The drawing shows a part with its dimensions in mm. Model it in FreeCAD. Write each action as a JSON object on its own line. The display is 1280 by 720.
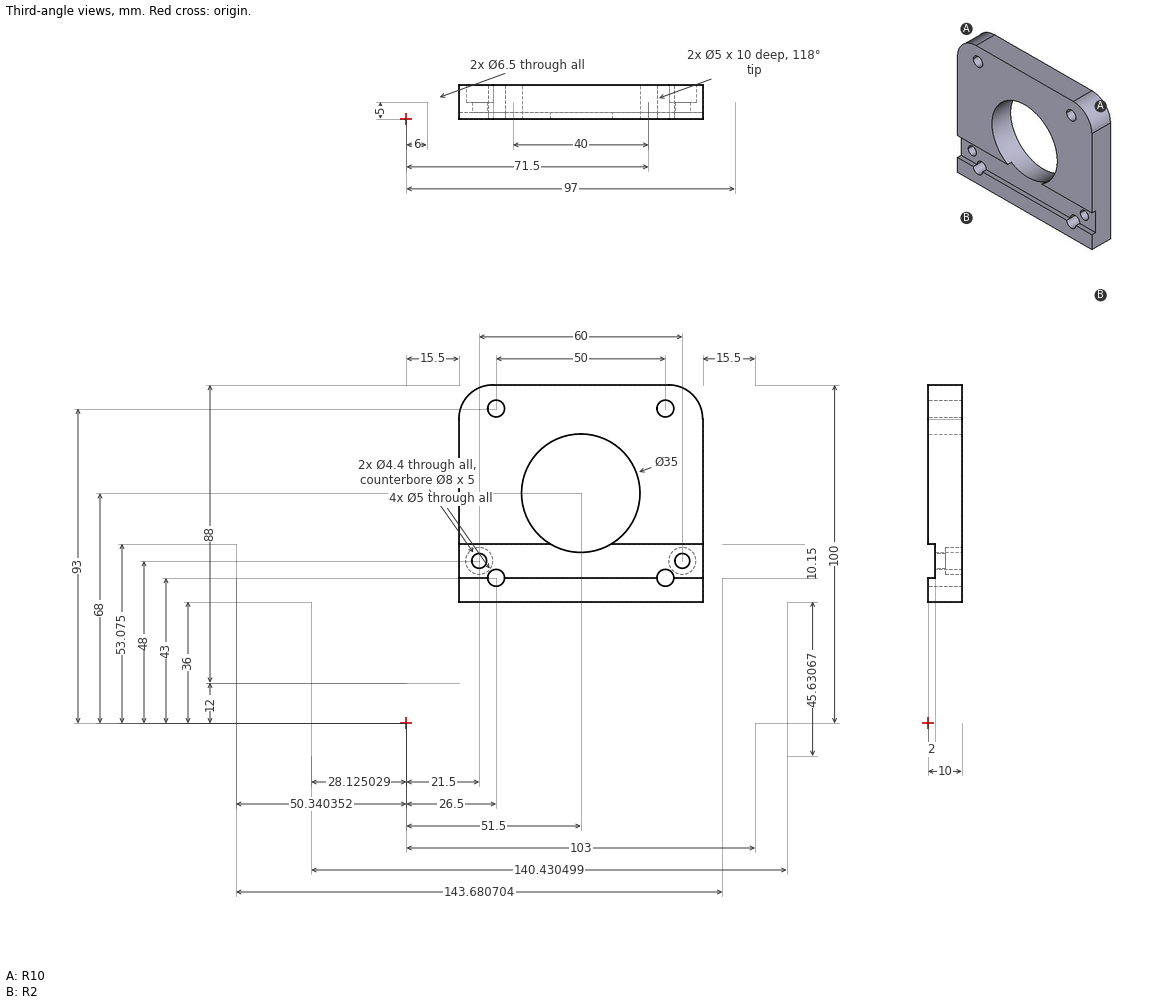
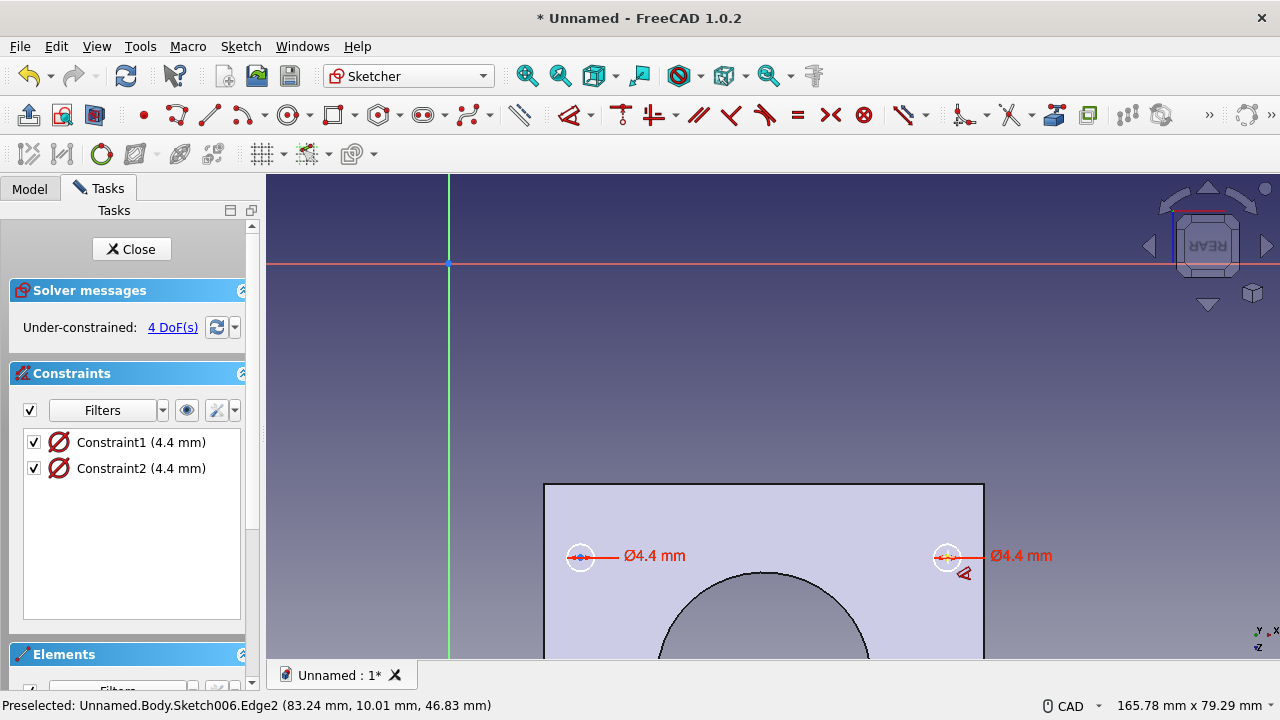
{"action": "left_click", "coordinate": [581, 558]}
{"action": "left_click", "coordinate": [415, 411]}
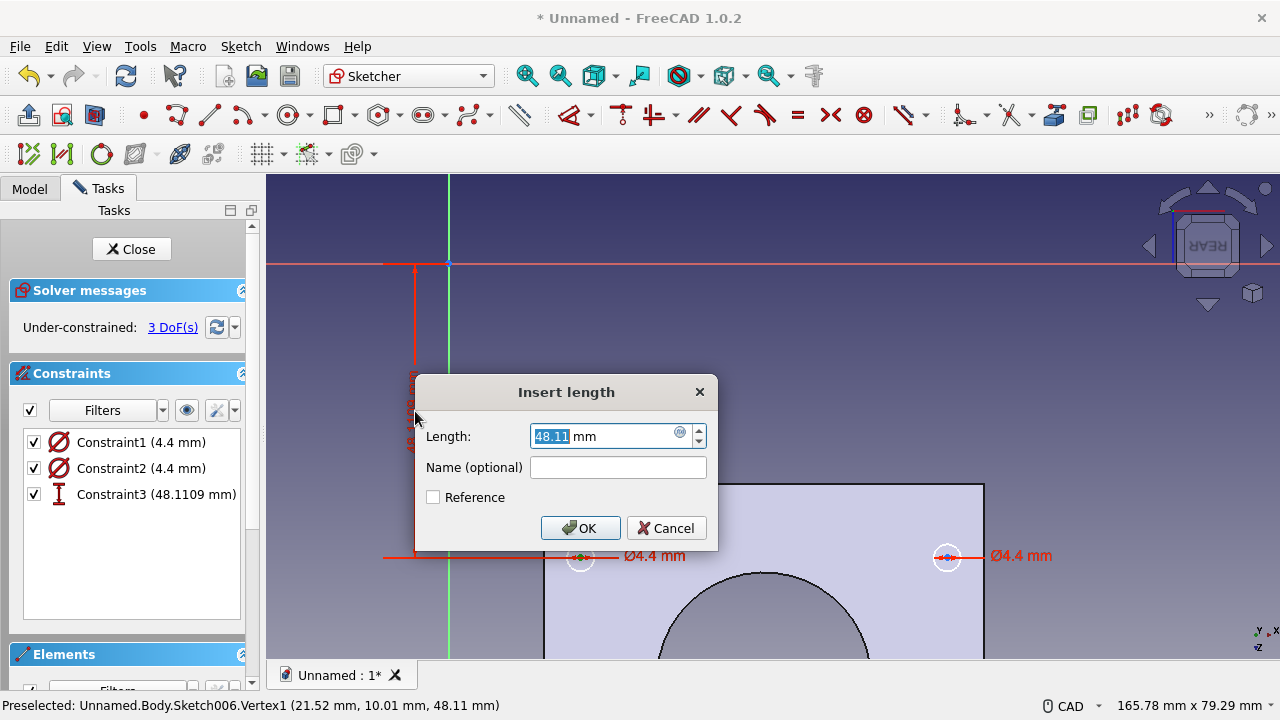
{"action": "type", "text": "48"}
{"action": "key", "text": "Return"}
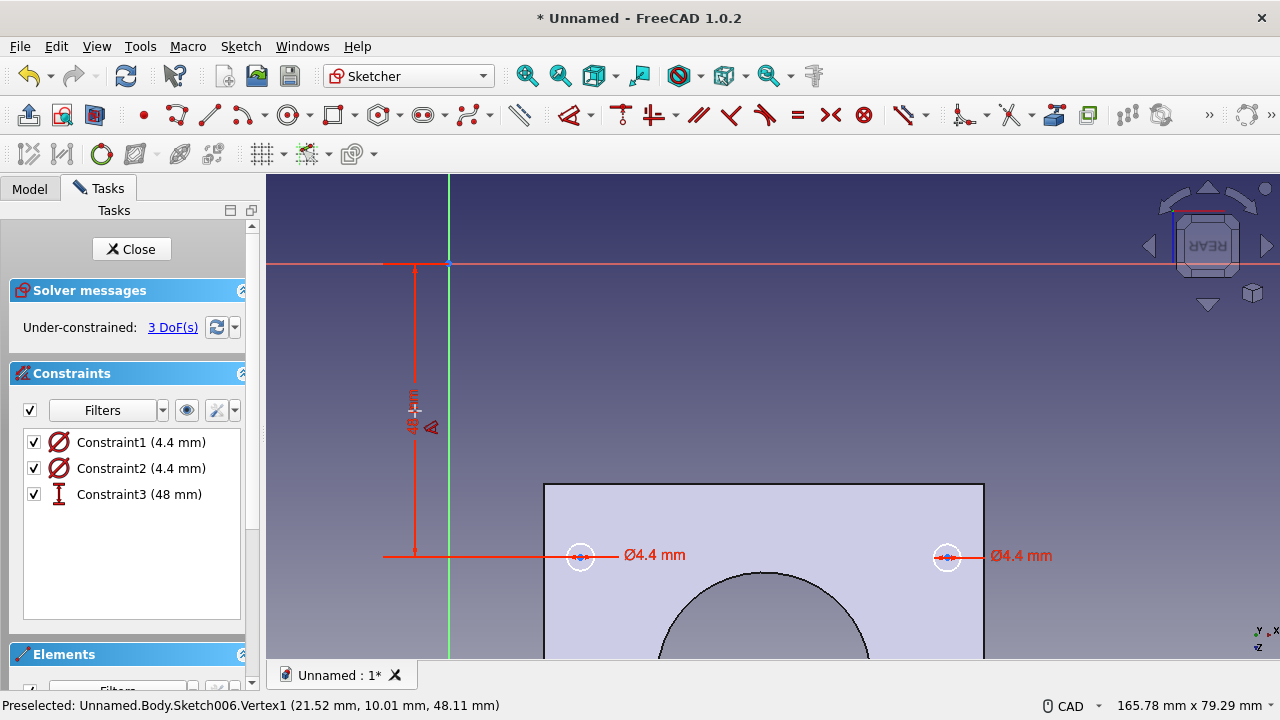
{"action": "left_click", "coordinate": [947, 558]}
{"action": "left_click", "coordinate": [415, 343]}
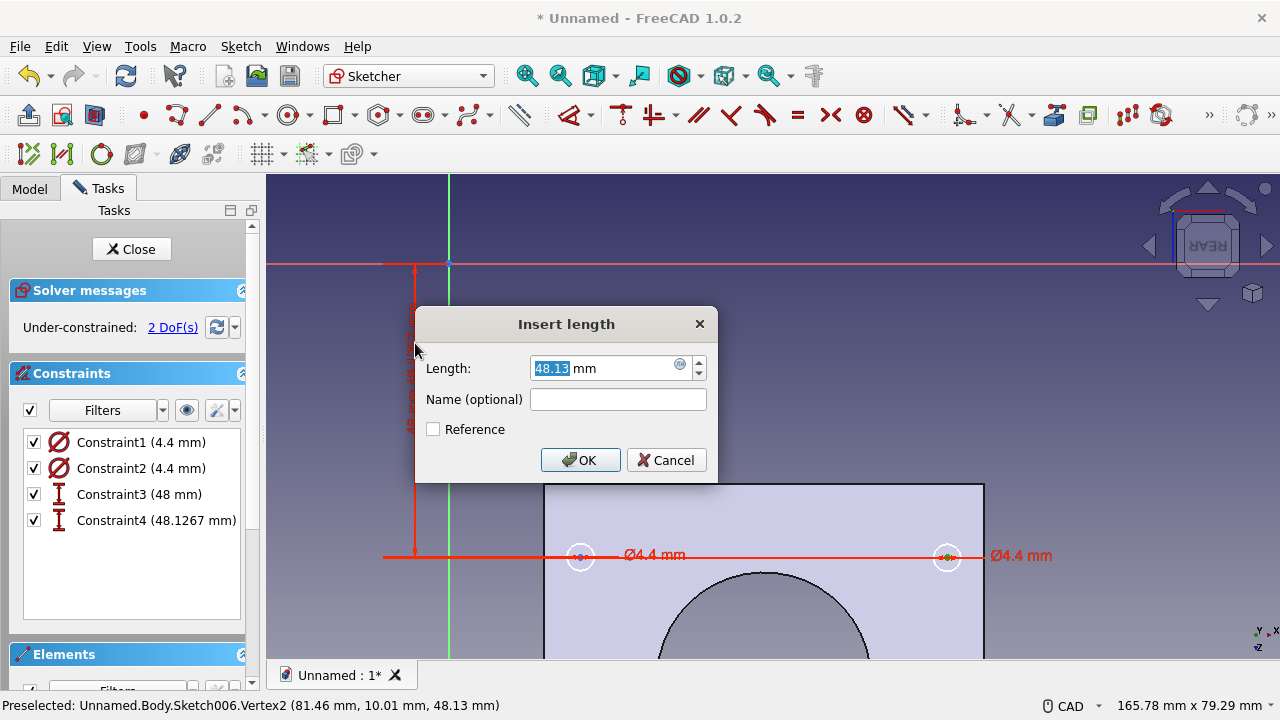
{"action": "type", "text": "48"}
{"action": "key", "text": "Return"}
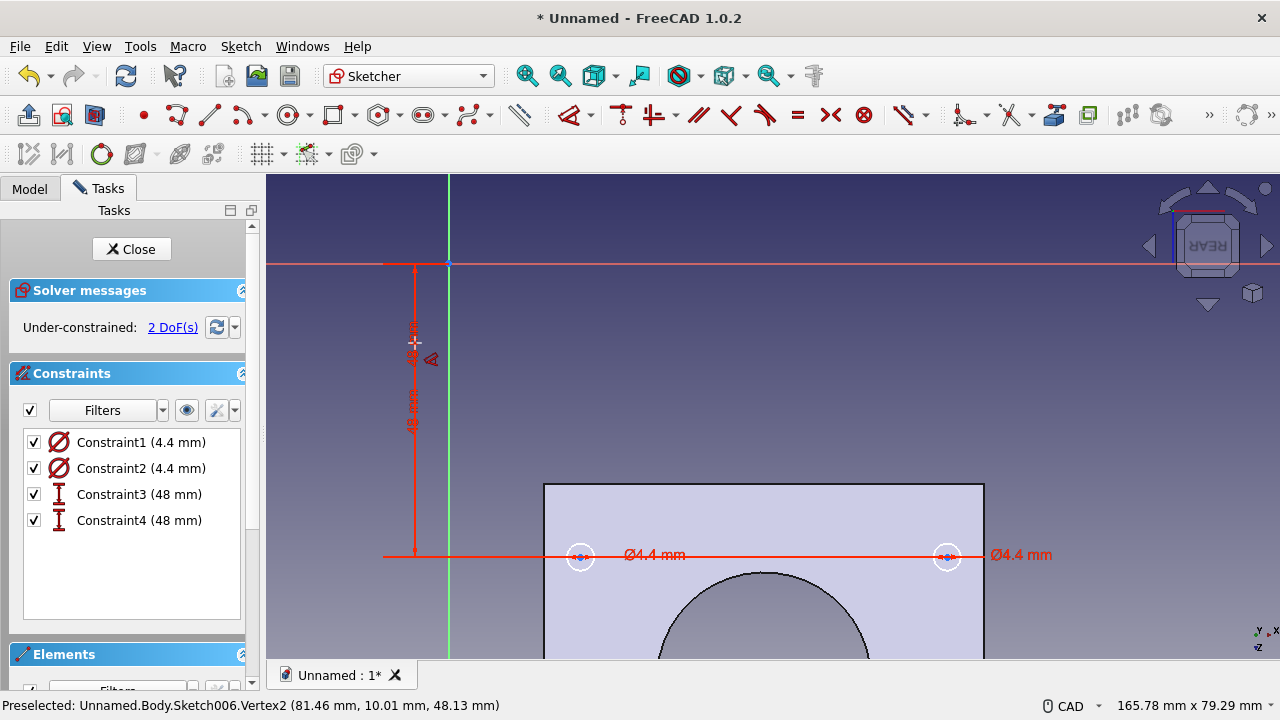
{"action": "left_click", "coordinate": [581, 557]}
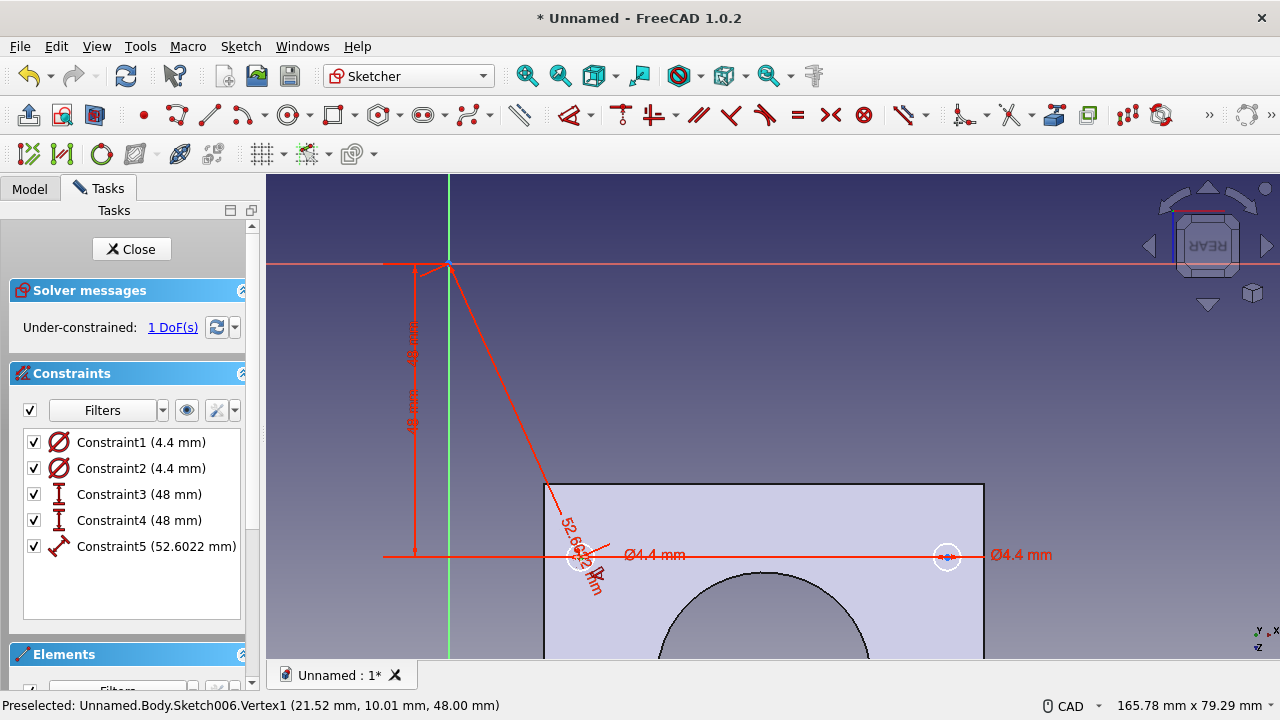
{"action": "left_click", "coordinate": [947, 557]}
{"action": "left_click", "coordinate": [764, 591]}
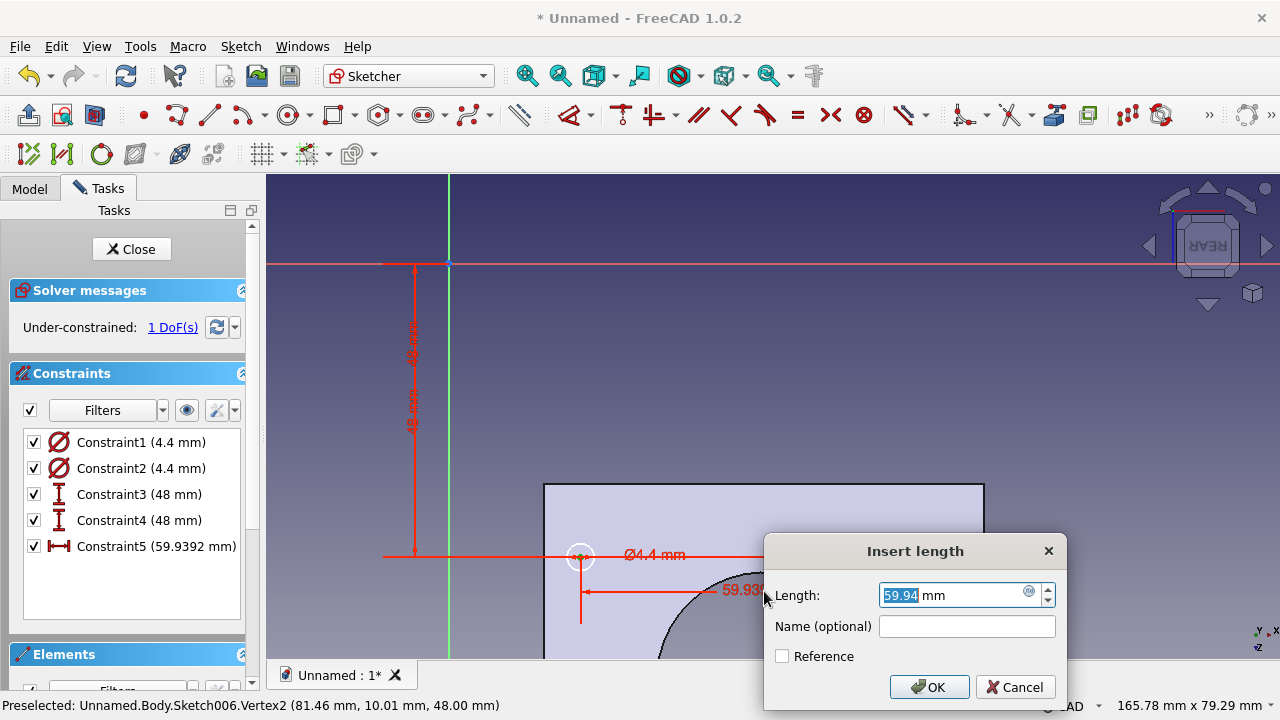
{"action": "type", "text": "60"}
{"action": "key", "text": "Return"}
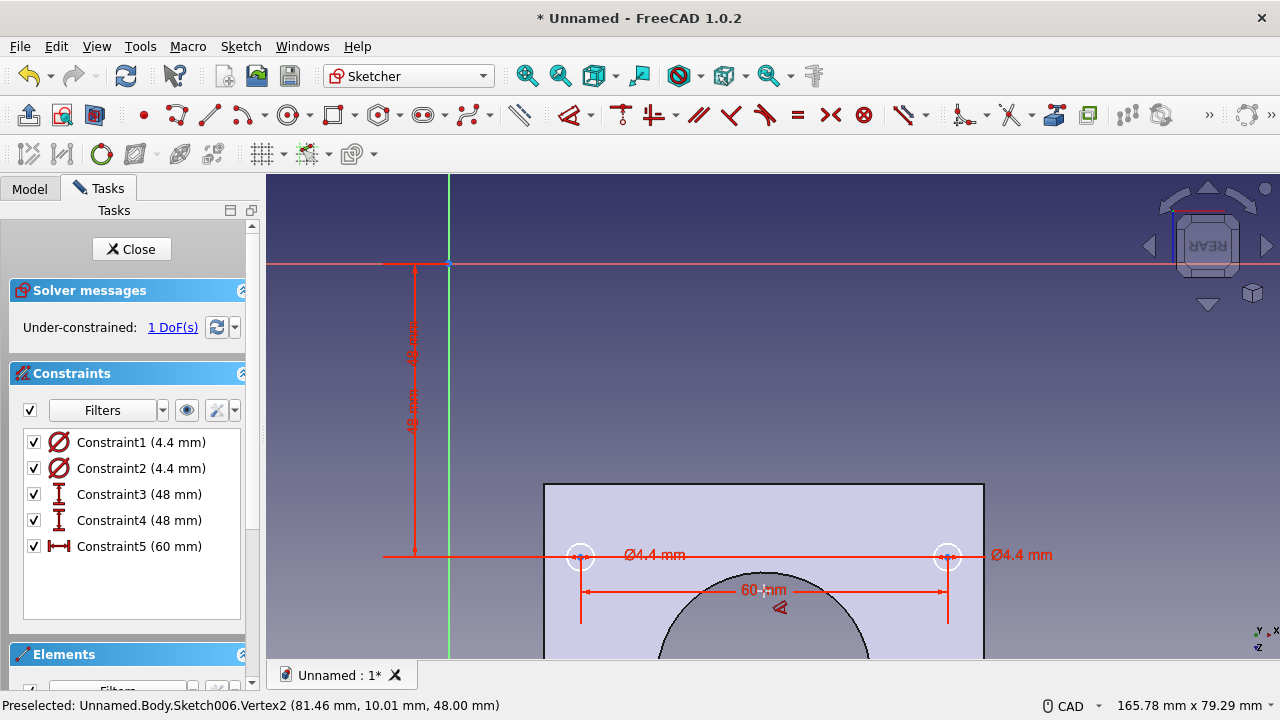
{"action": "left_click", "coordinate": [581, 557]}
{"action": "left_click", "coordinate": [515, 230]}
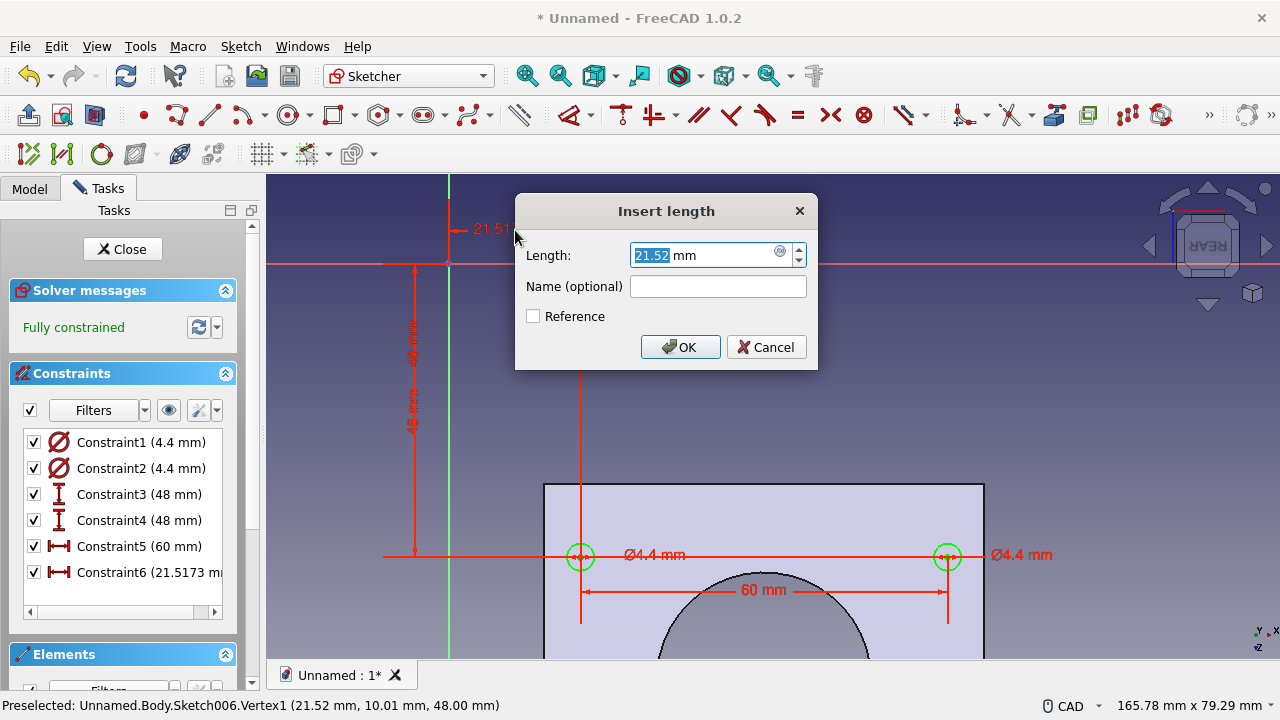
{"action": "type", "text": "21.5"}
{"action": "key", "text": "Return"}
{"action": "key", "text": "Escape"}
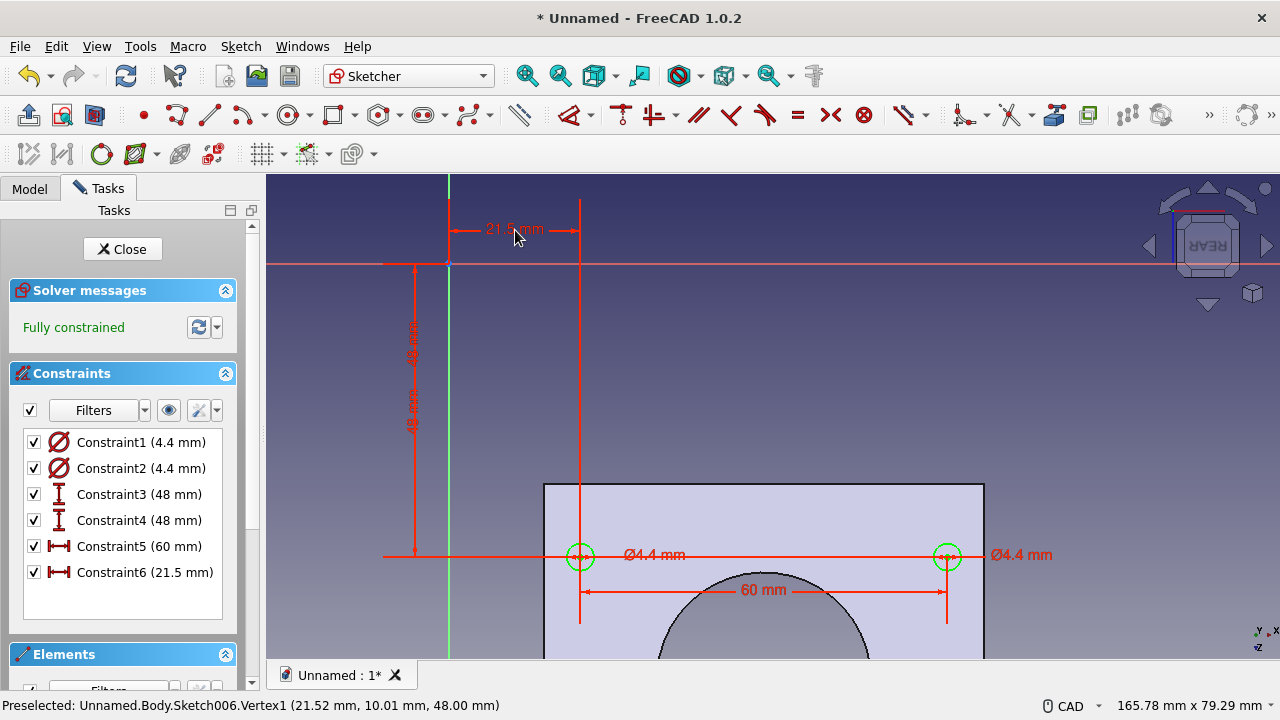
{"action": "left_click", "coordinate": [123, 249]}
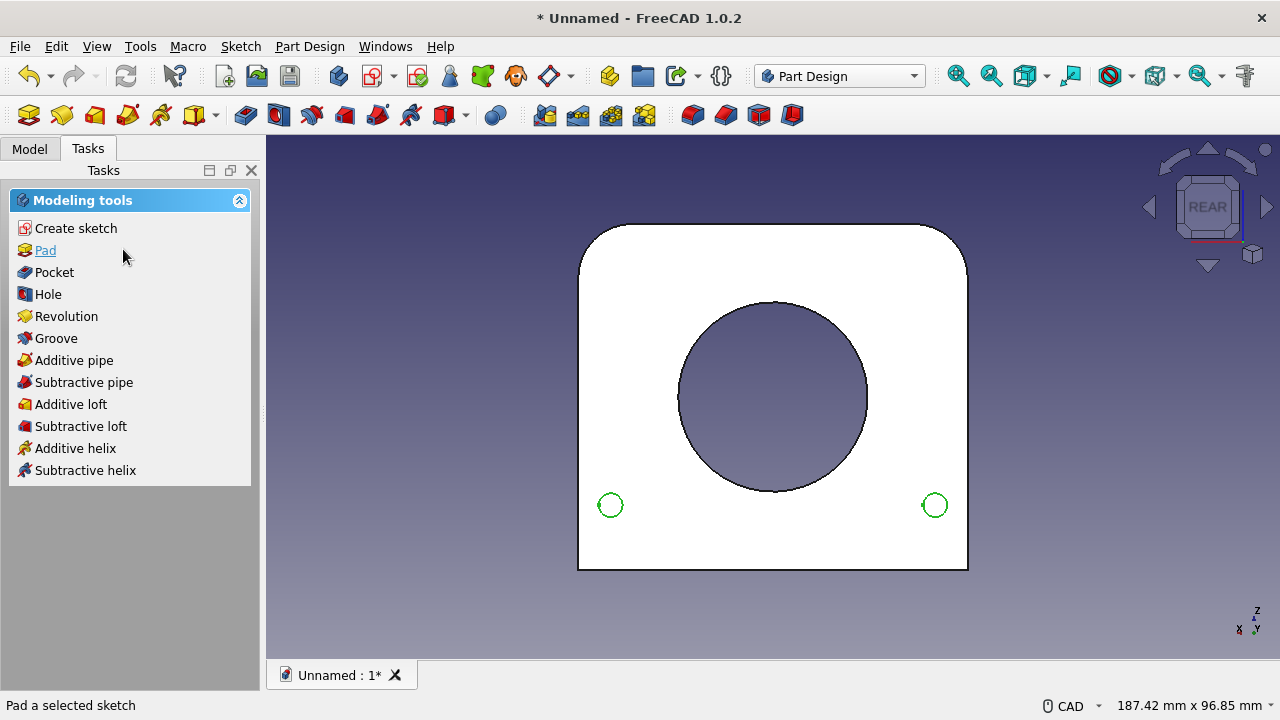
{"action": "left_click", "coordinate": [279, 116]}